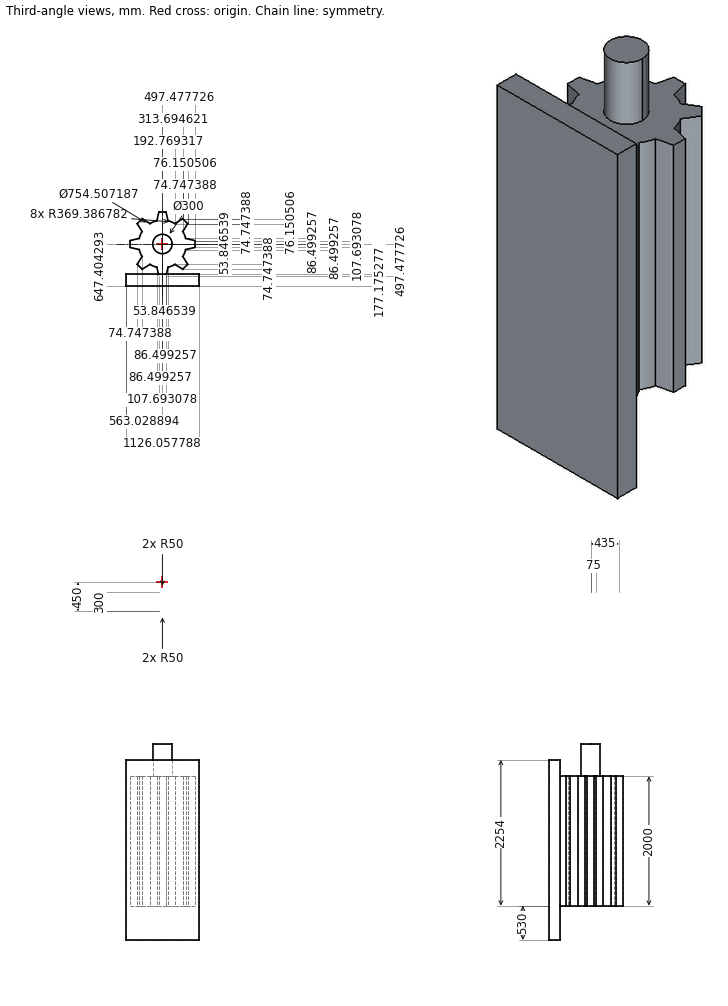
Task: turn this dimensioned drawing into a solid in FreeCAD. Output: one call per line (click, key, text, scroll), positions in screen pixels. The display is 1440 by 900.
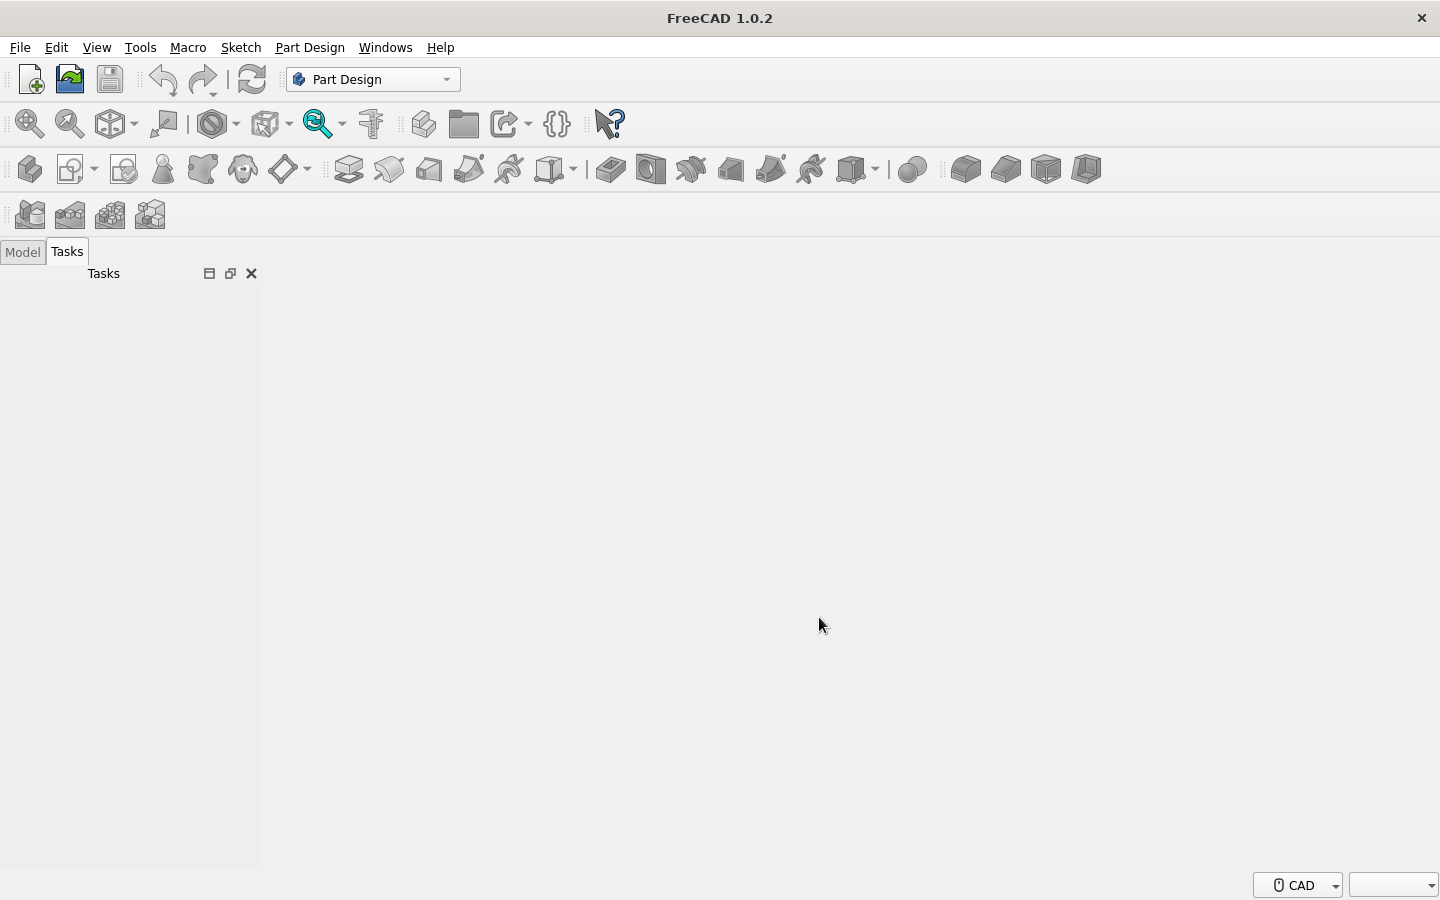
click(30, 80)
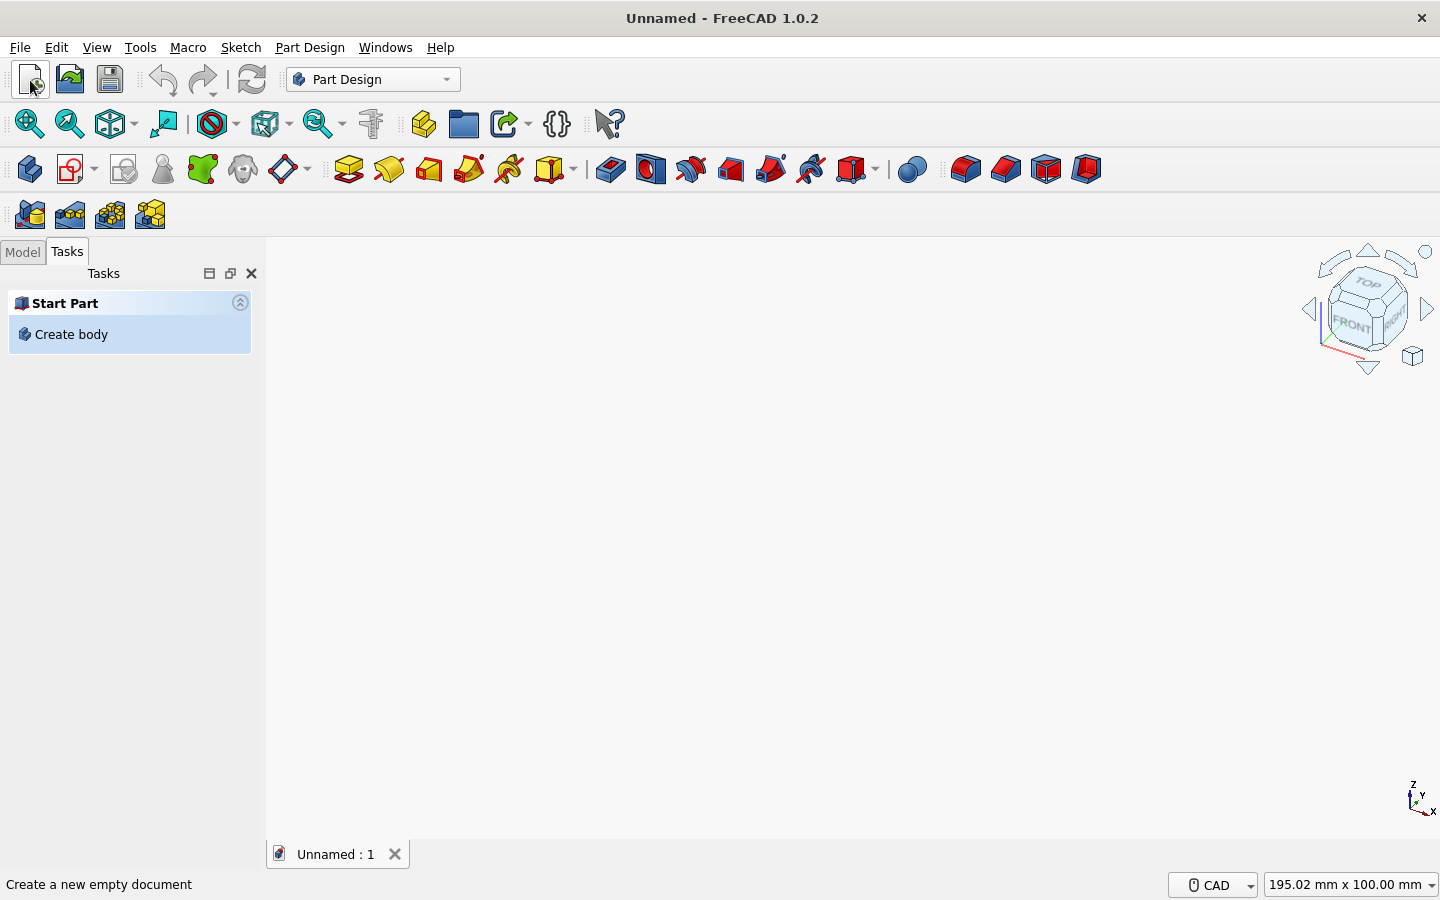
click(70, 170)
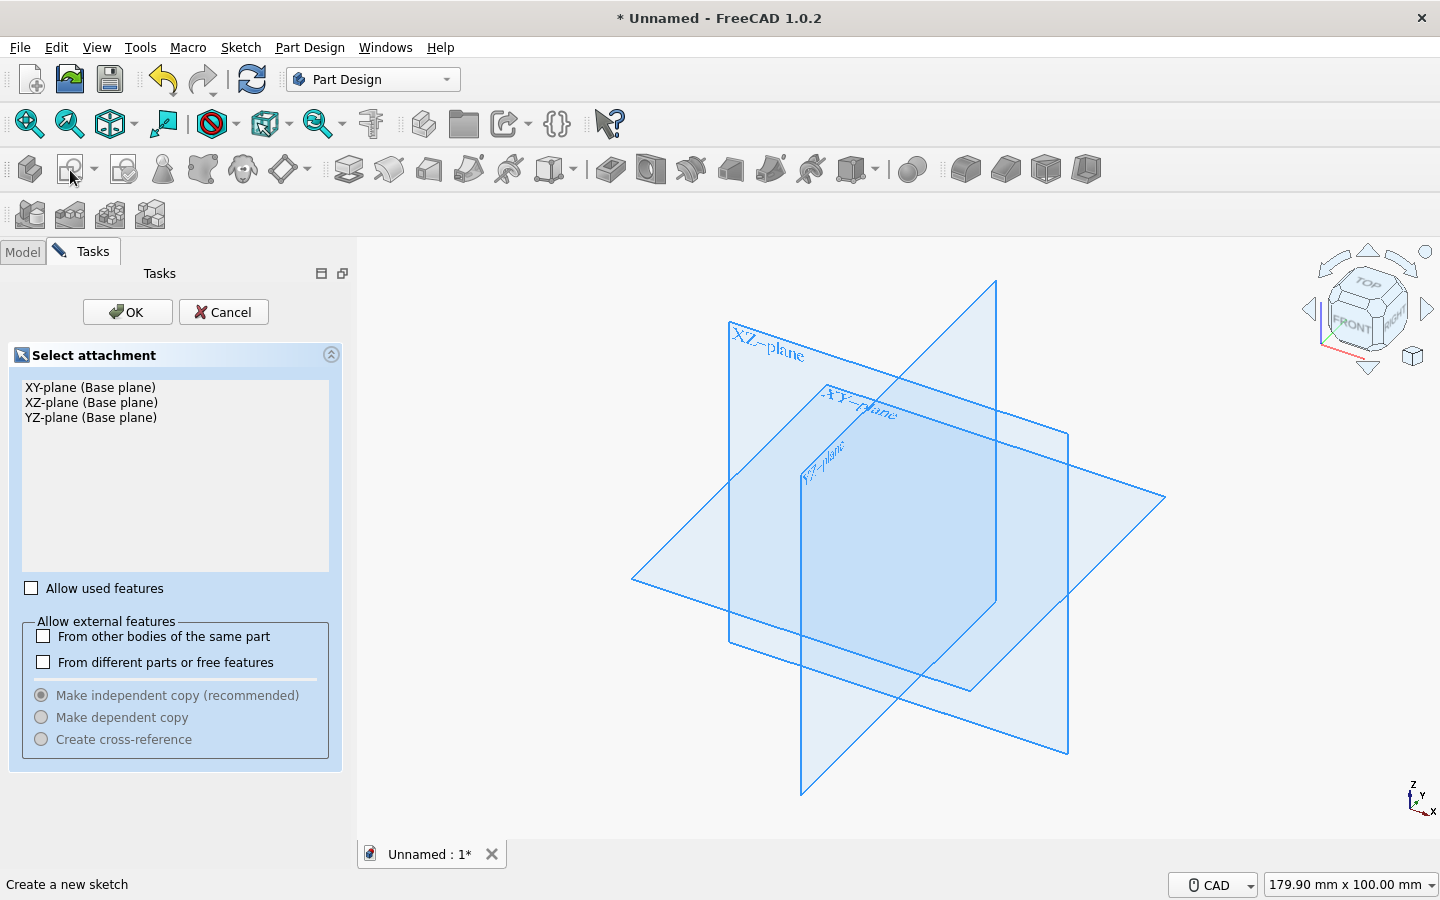
click(82, 388)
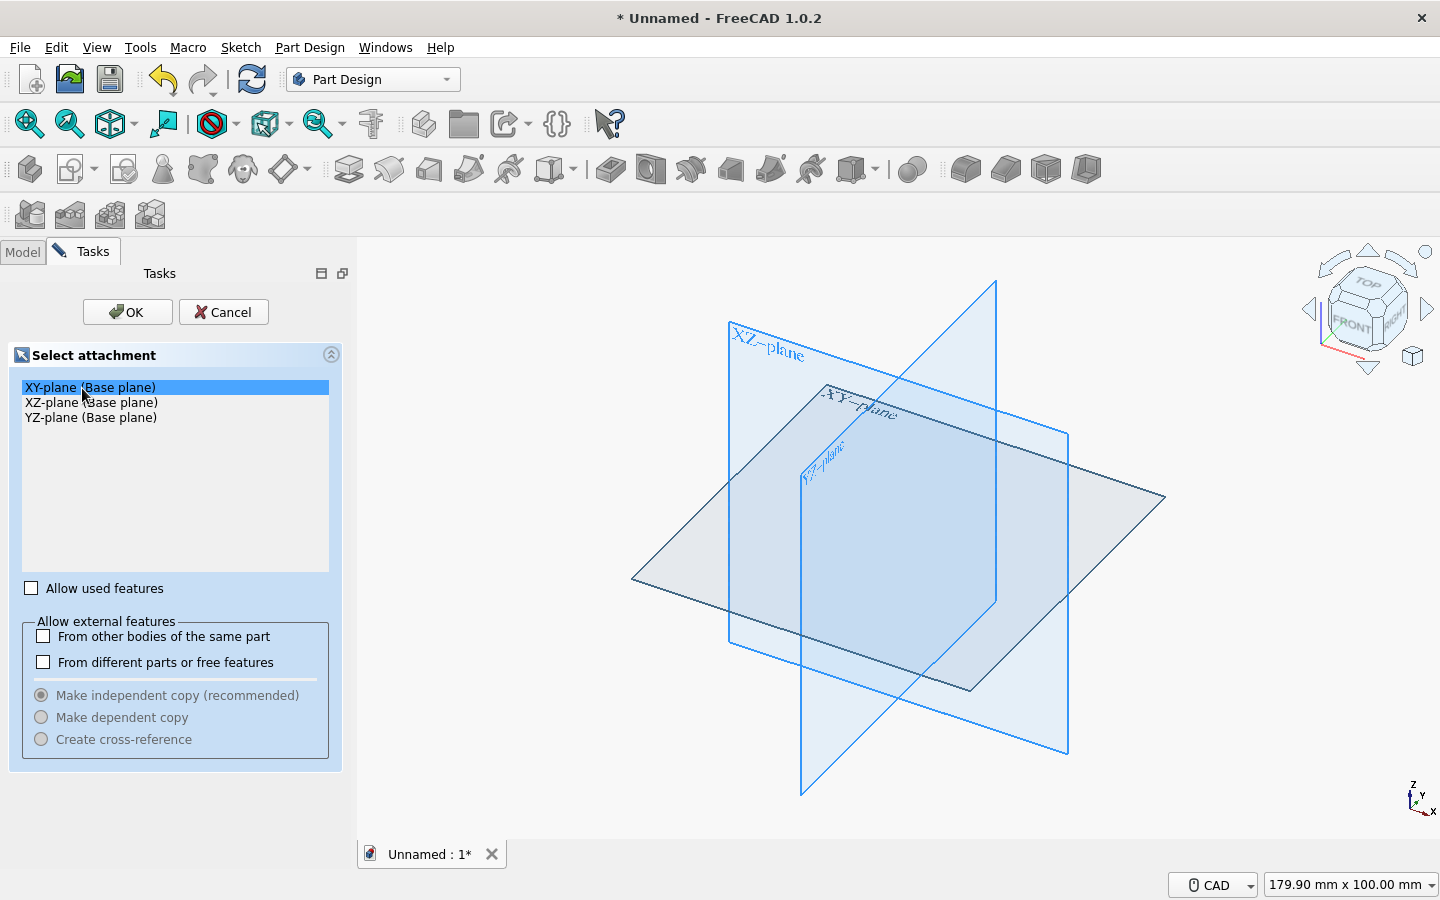
click(128, 312)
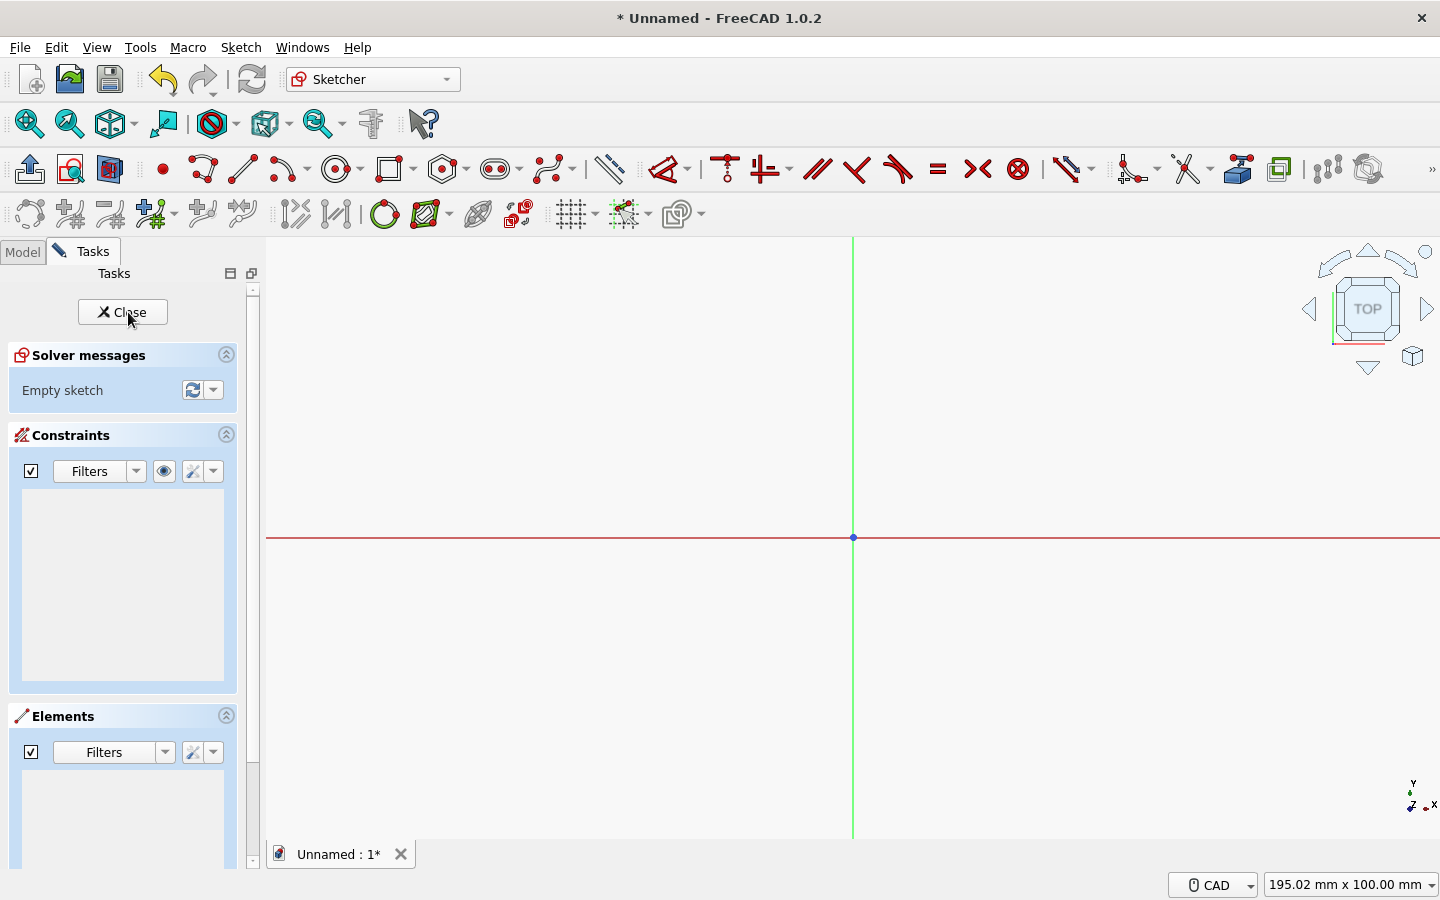
scroll(767, 538, down, 8)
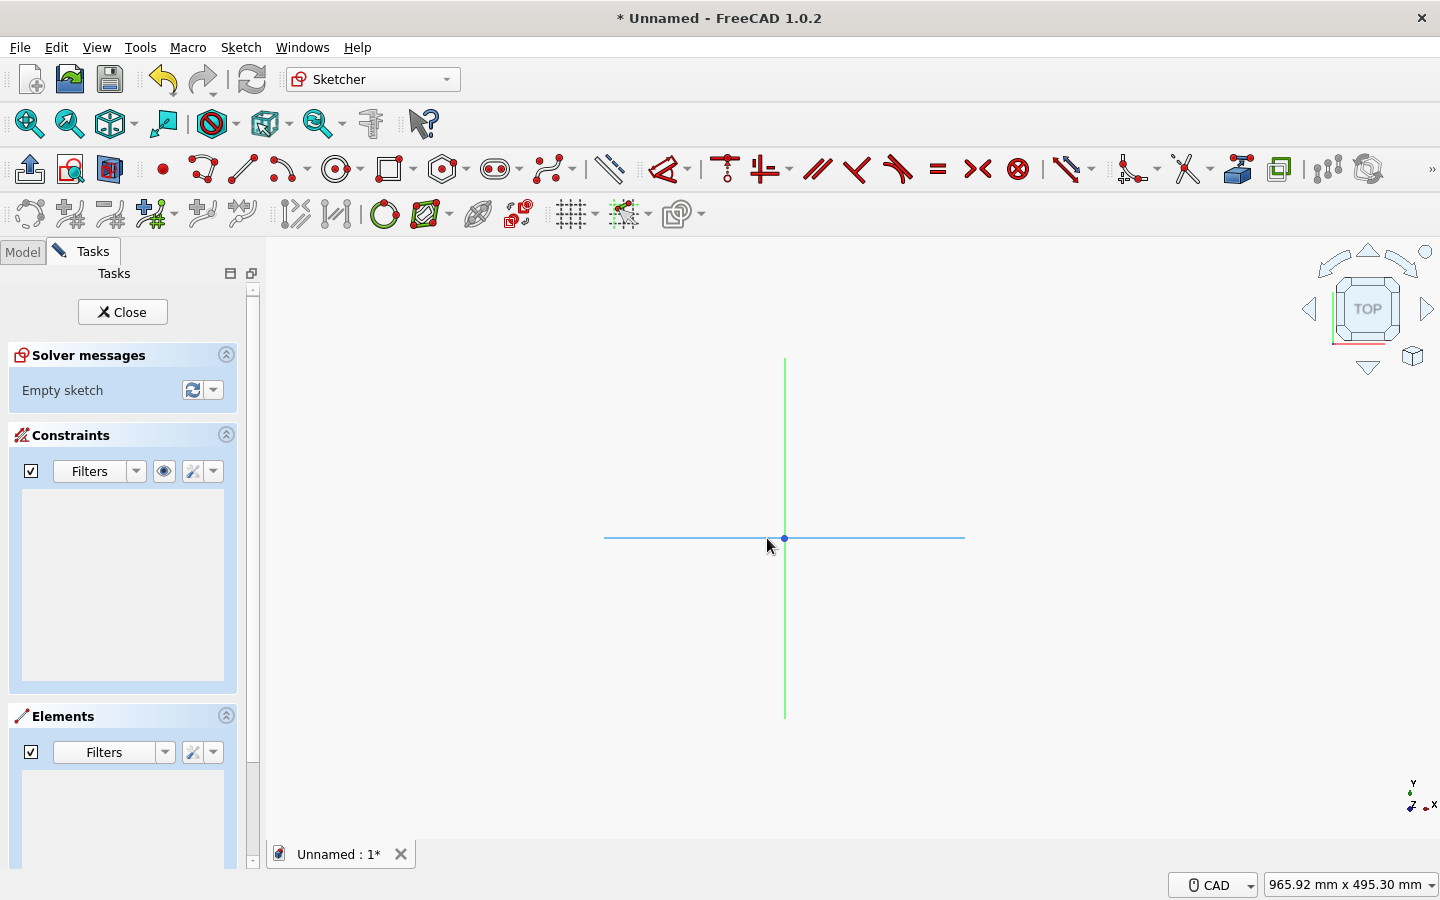
click(336, 170)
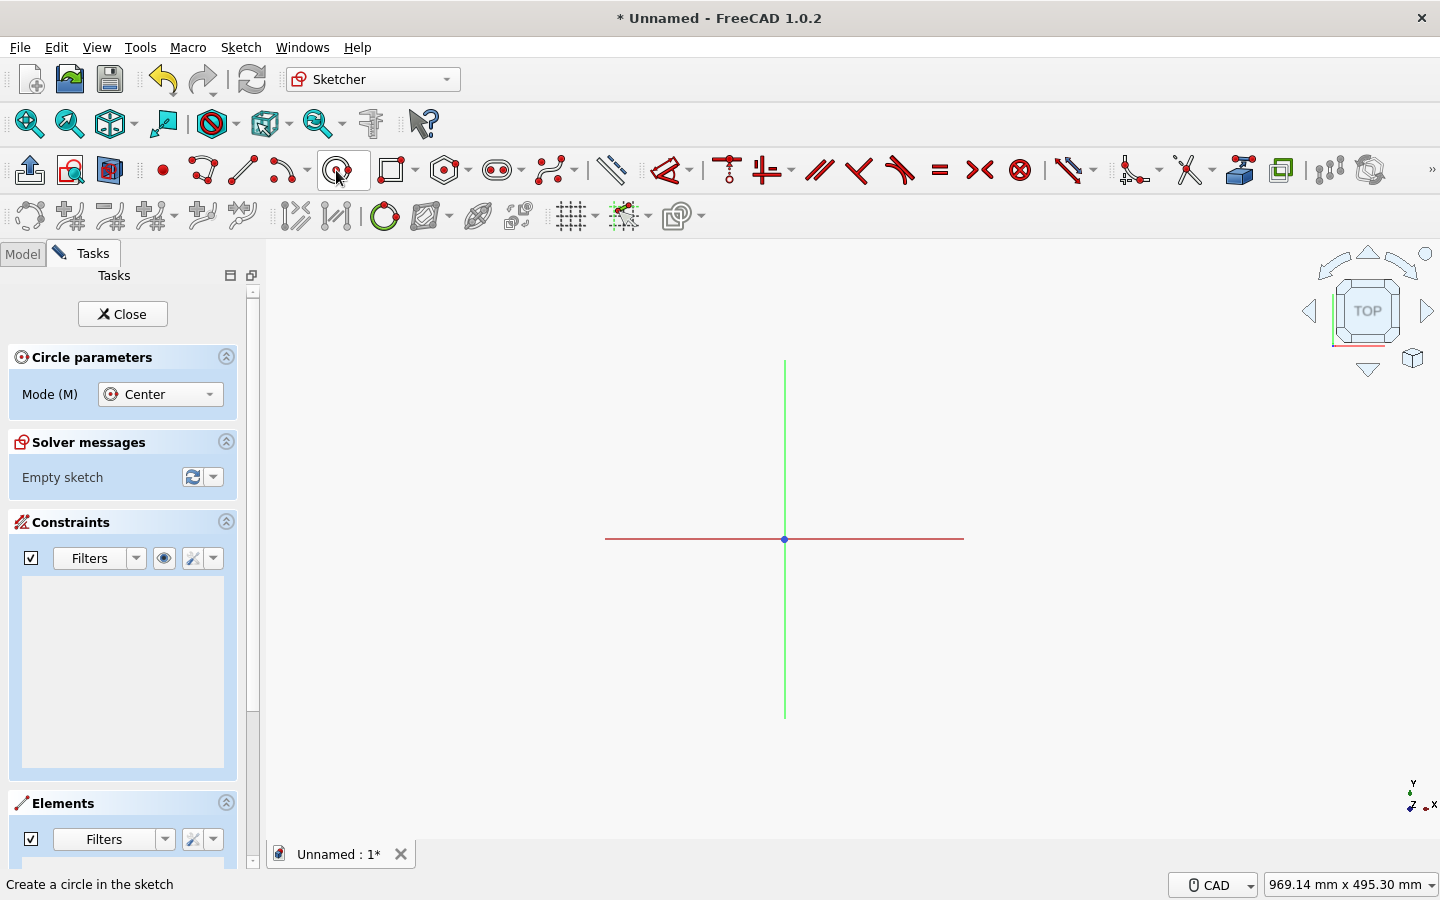
click(785, 539)
move(913, 411)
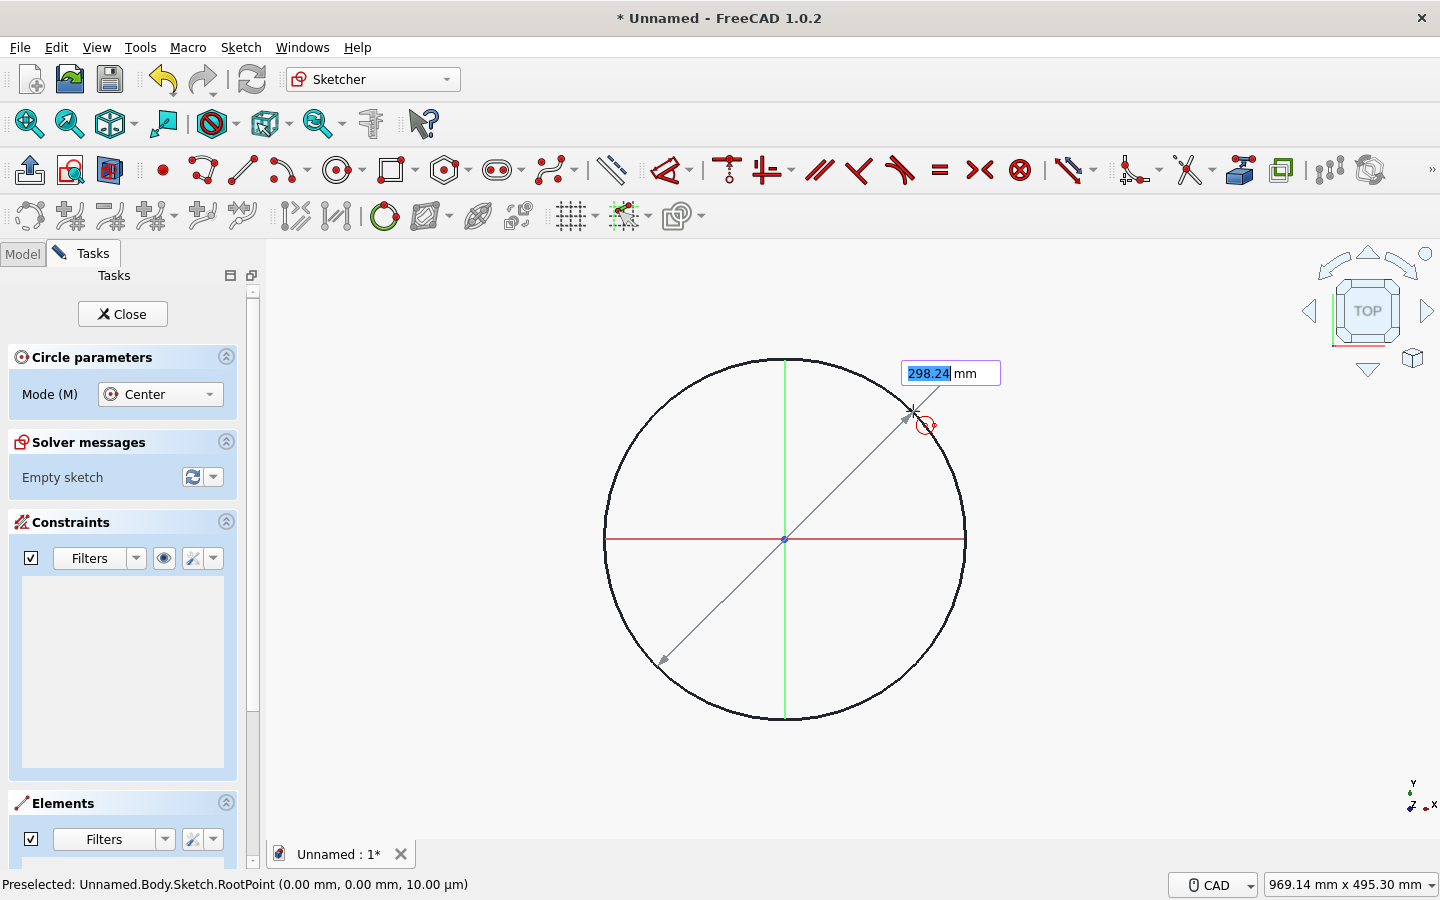
text(300)
key(Return)
key(Escape)